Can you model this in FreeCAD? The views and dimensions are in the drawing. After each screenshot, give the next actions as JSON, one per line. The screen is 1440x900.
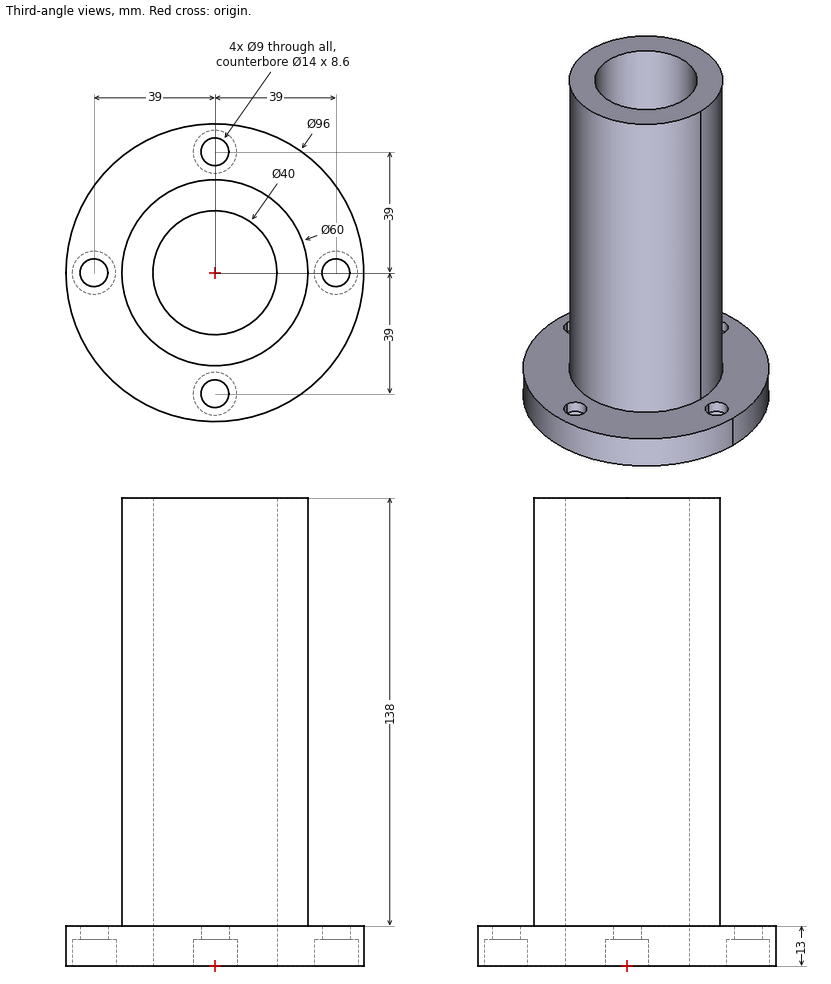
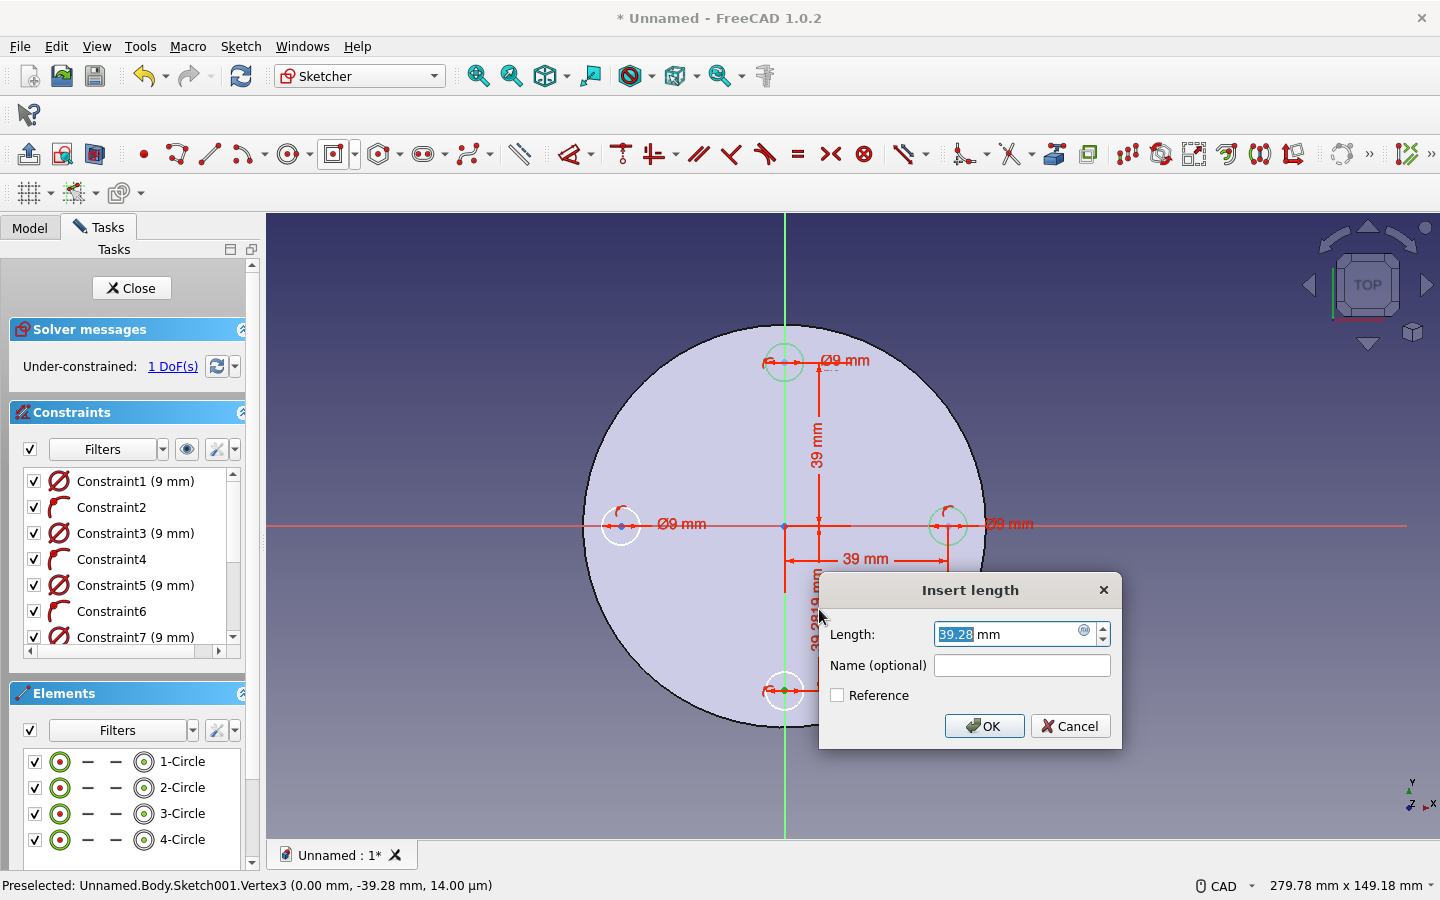
{"action": "type", "text": "39"}
{"action": "key", "text": "Return"}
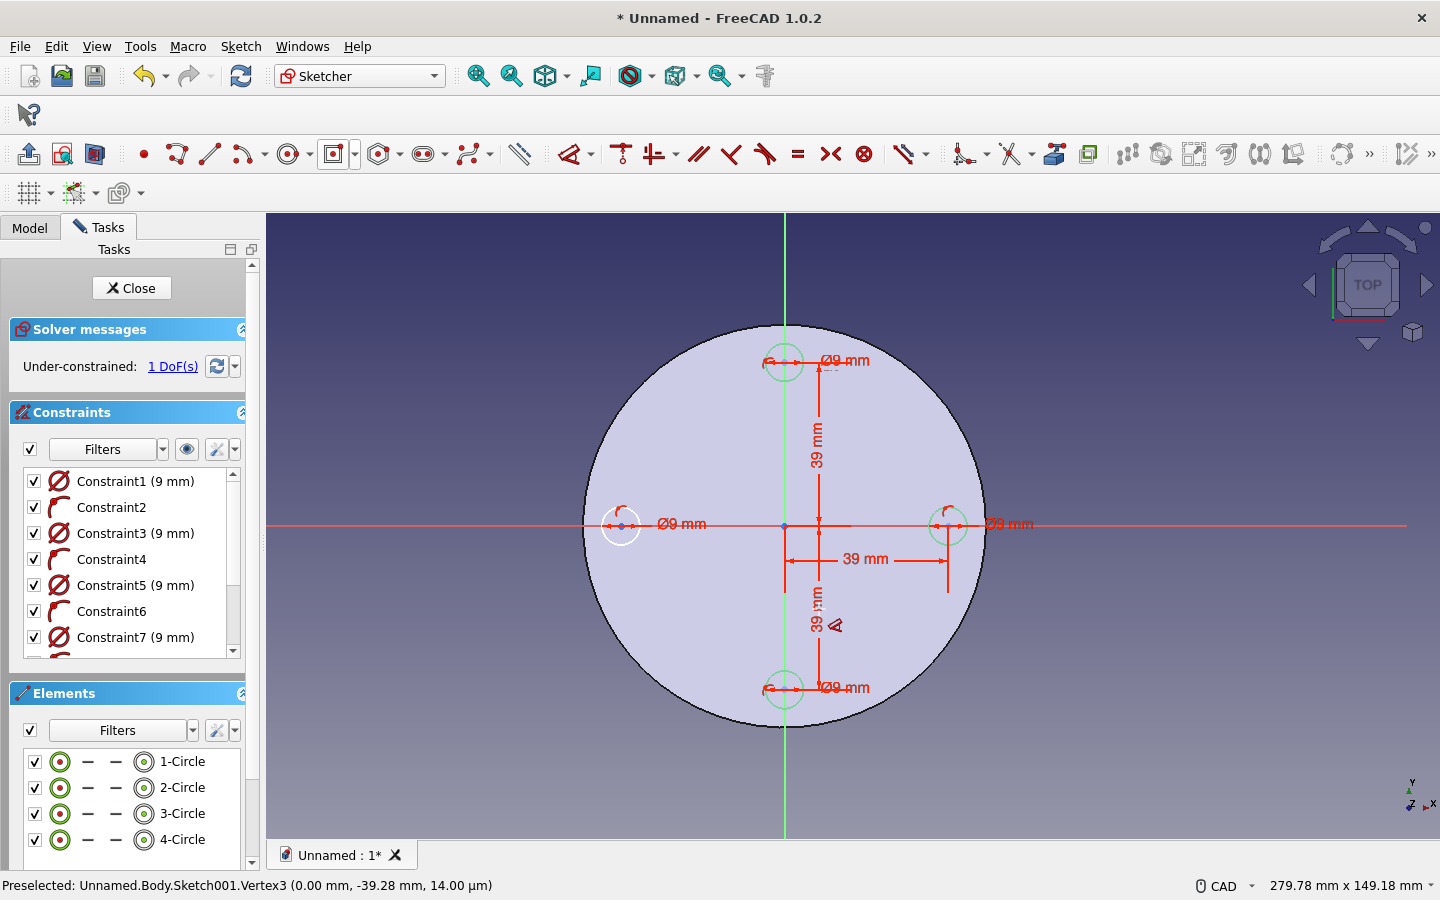
{"action": "left_click", "coordinate": [621, 526]}
{"action": "left_click", "coordinate": [703, 560]}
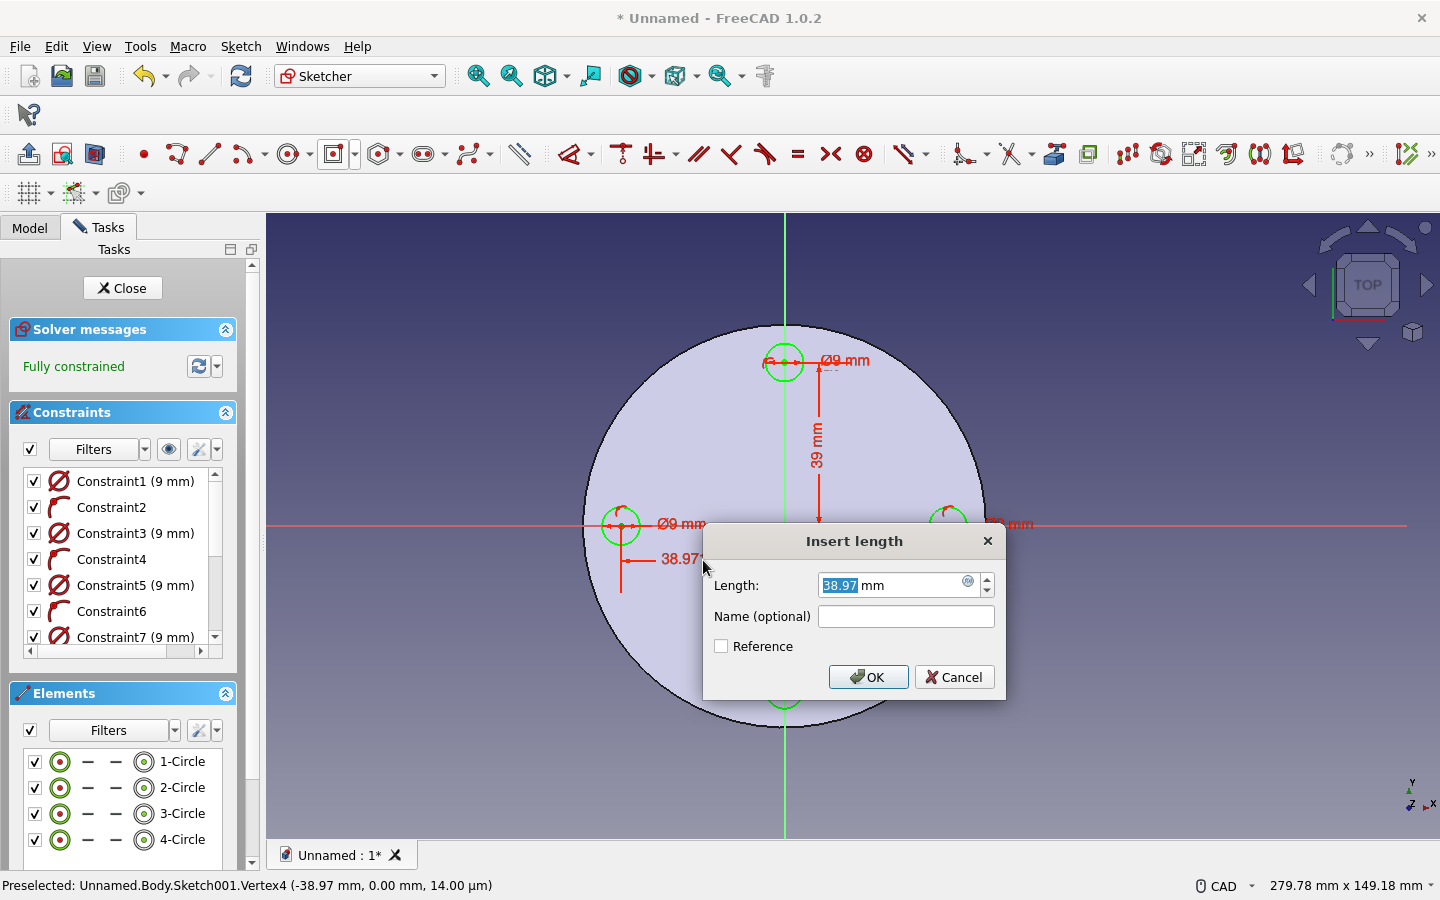
{"action": "type", "text": "39"}
{"action": "key", "text": "Return"}
{"action": "key", "text": "Escape"}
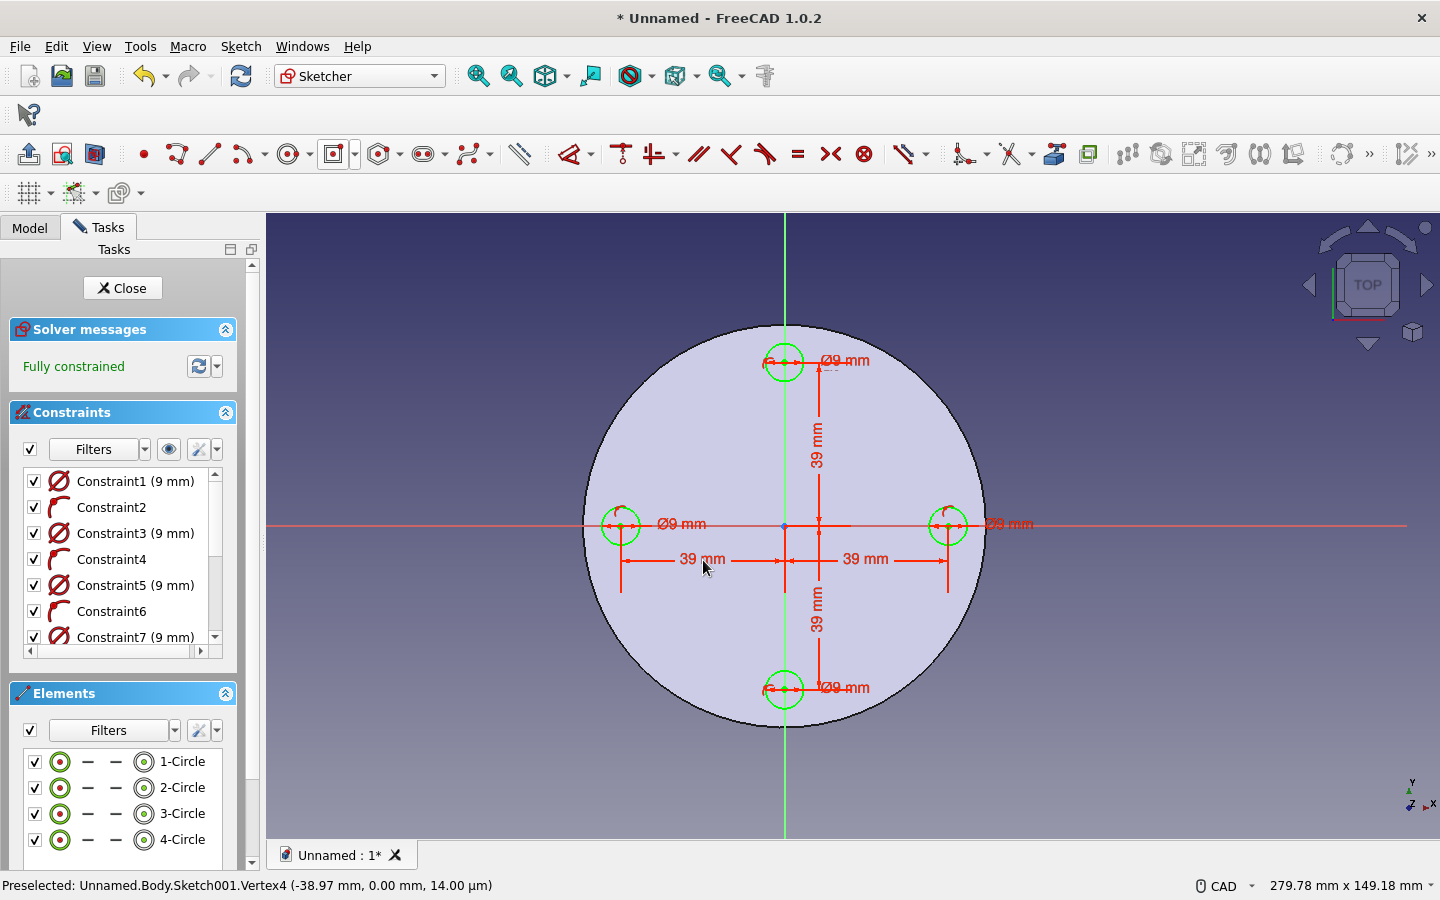
{"action": "left_click", "coordinate": [123, 288]}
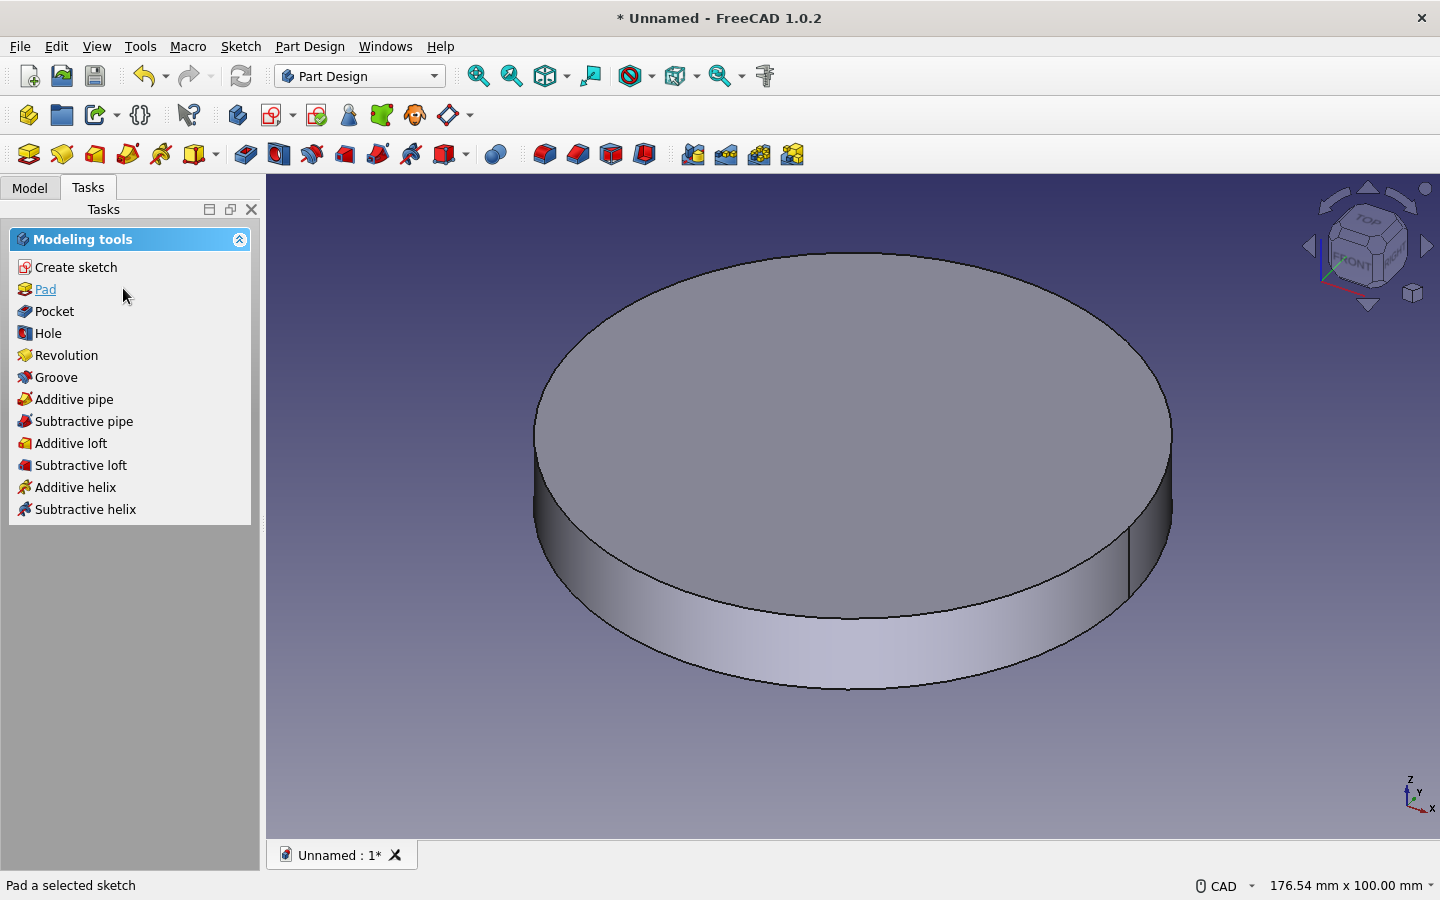
{"action": "left_click", "coordinate": [279, 154]}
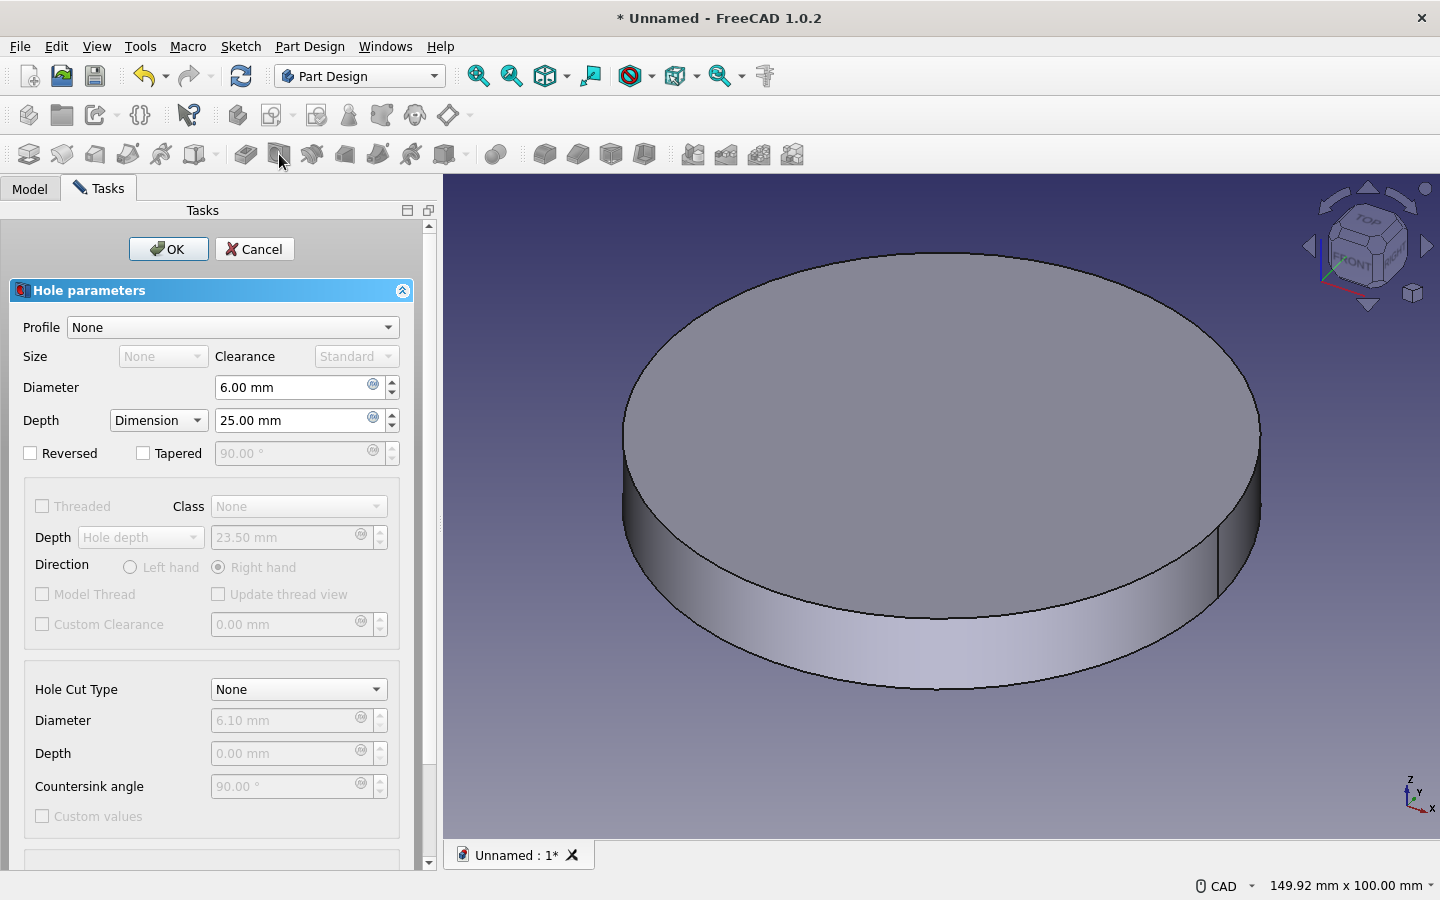
{"action": "triple_click", "coordinate": [300, 388]}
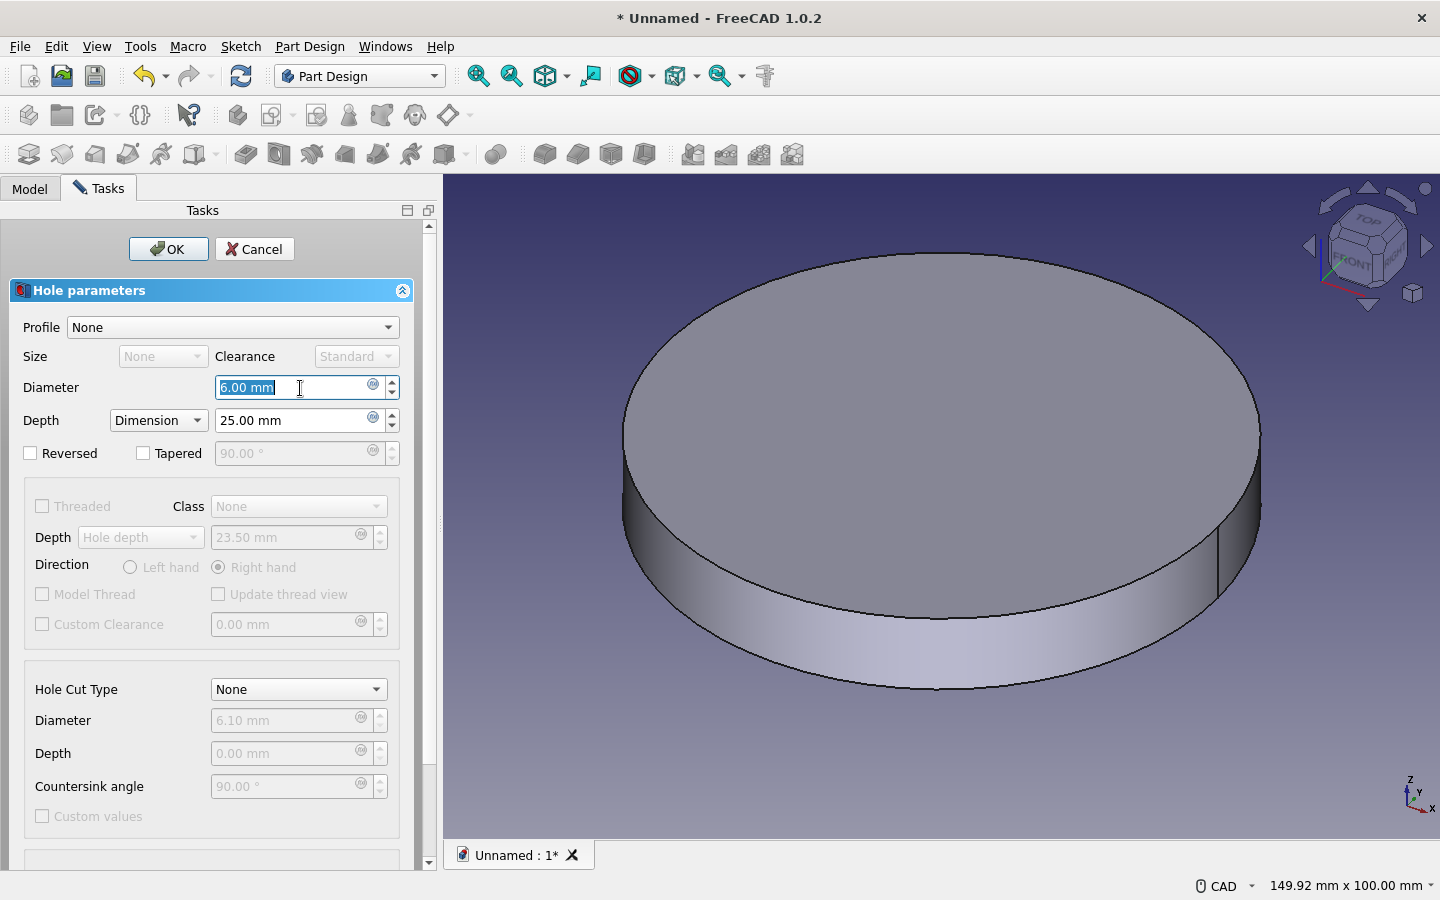
{"action": "type", "text": "9"}
{"action": "key", "text": "Tab"}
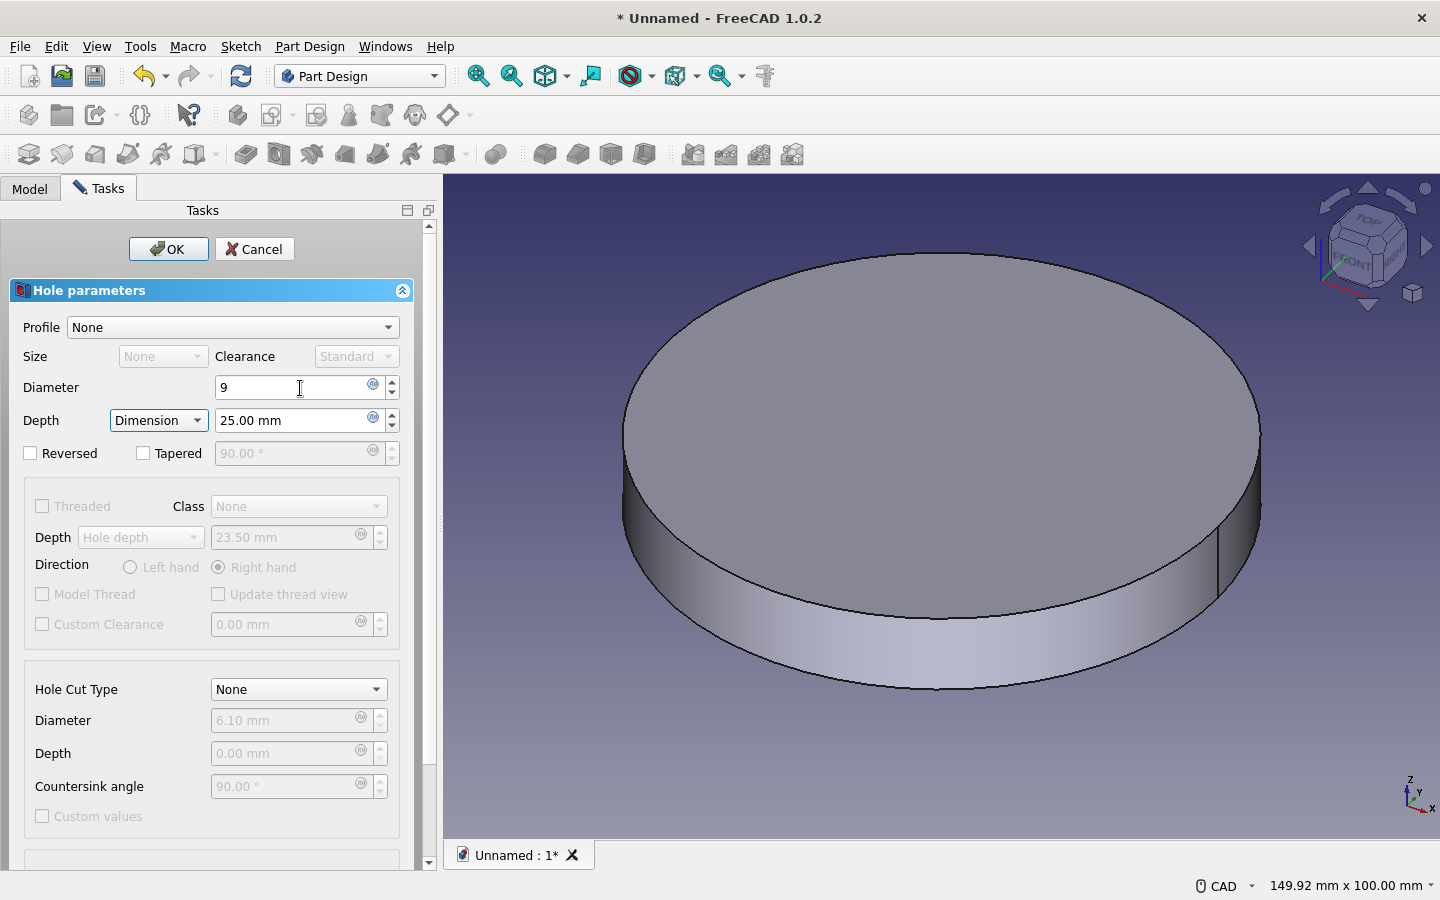
{"action": "left_click", "coordinate": [160, 420]}